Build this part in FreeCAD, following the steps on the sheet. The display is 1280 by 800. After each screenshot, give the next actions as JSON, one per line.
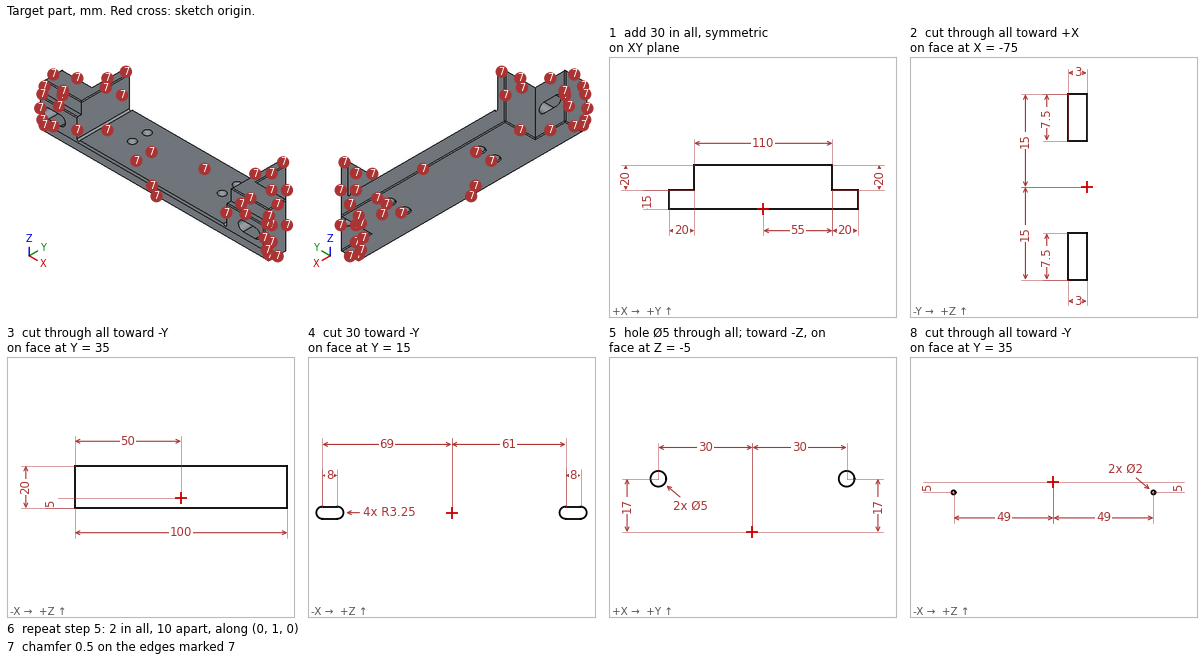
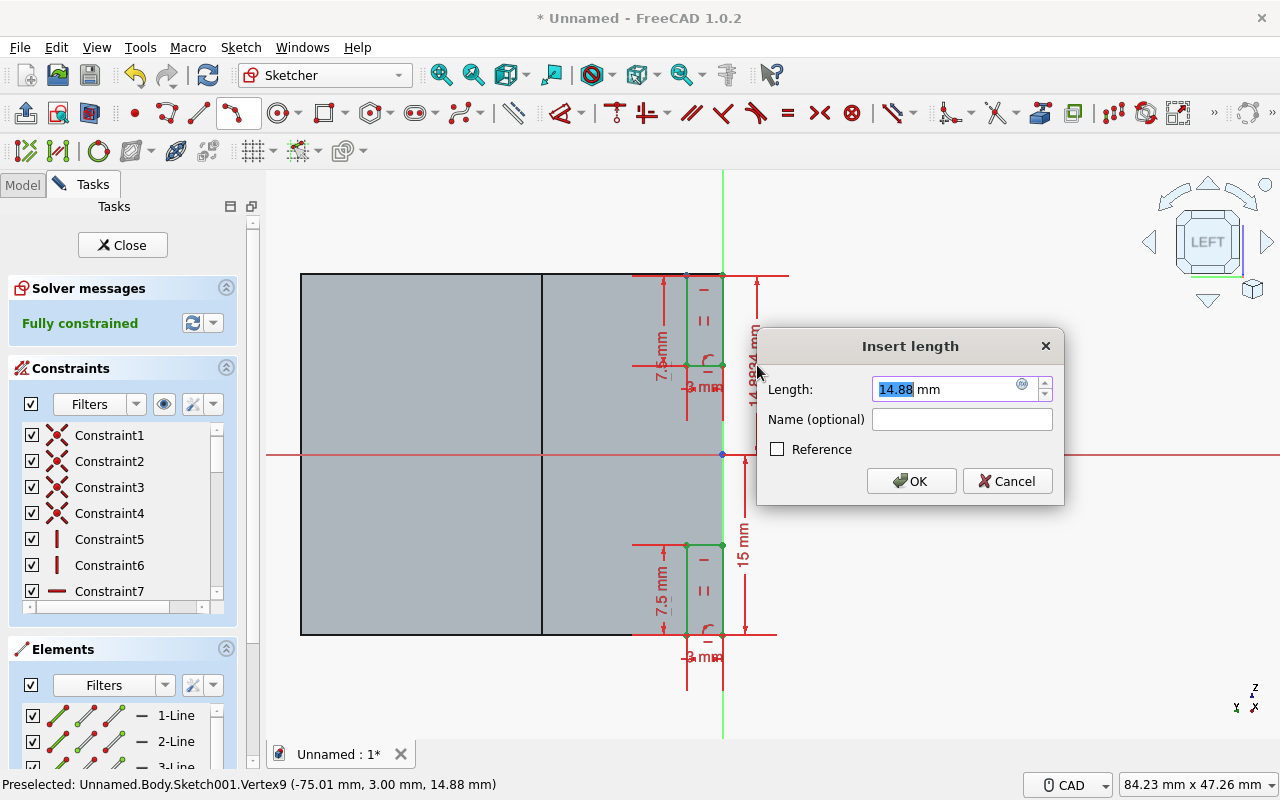
{"action": "type", "text": "15"}
{"action": "key", "text": "Return"}
{"action": "key", "text": "Escape"}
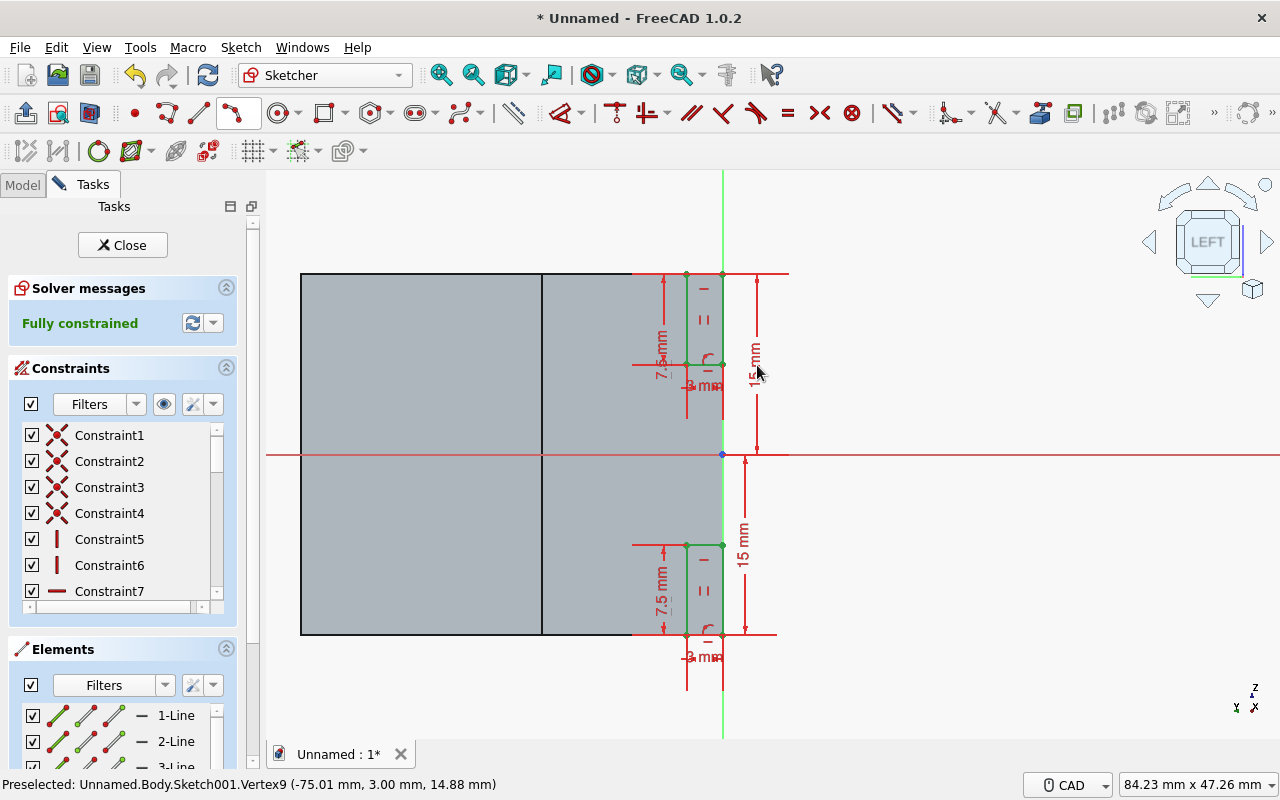
{"action": "left_click", "coordinate": [123, 245]}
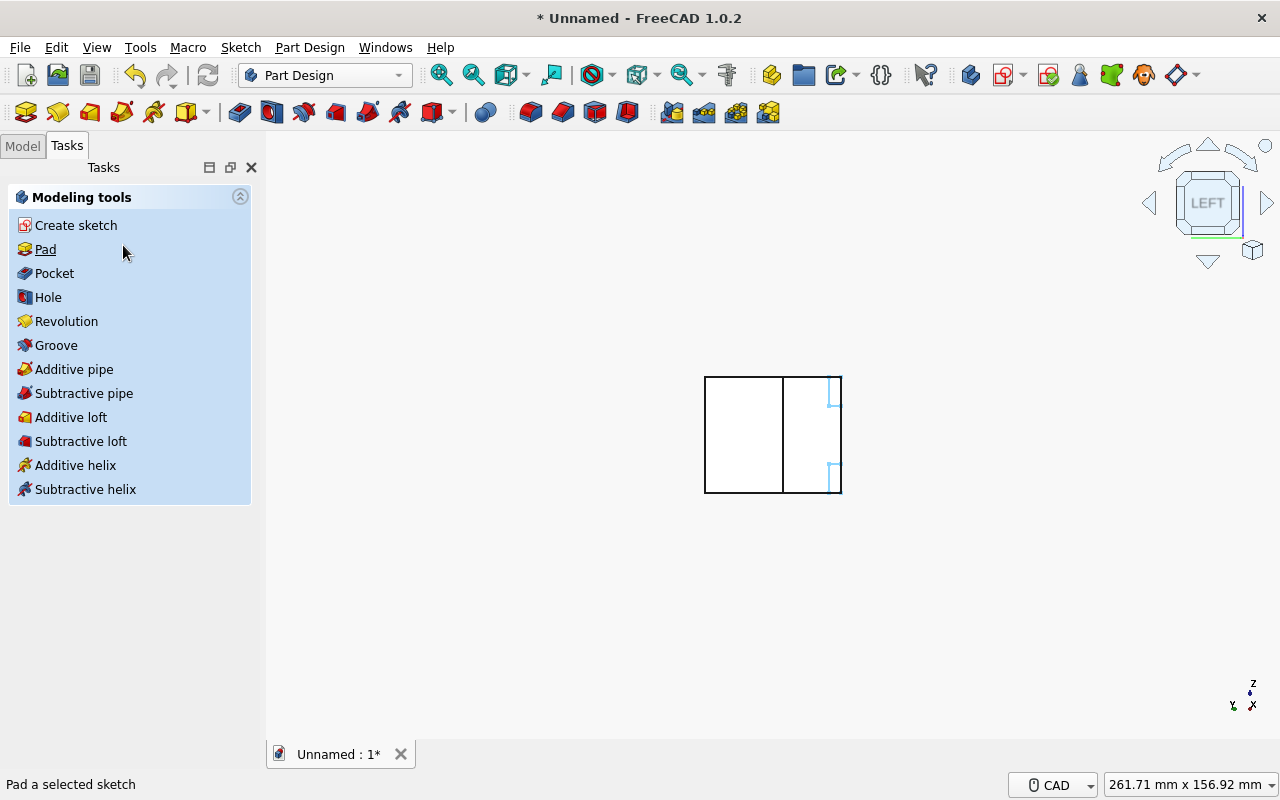
{"action": "left_click", "coordinate": [240, 112]}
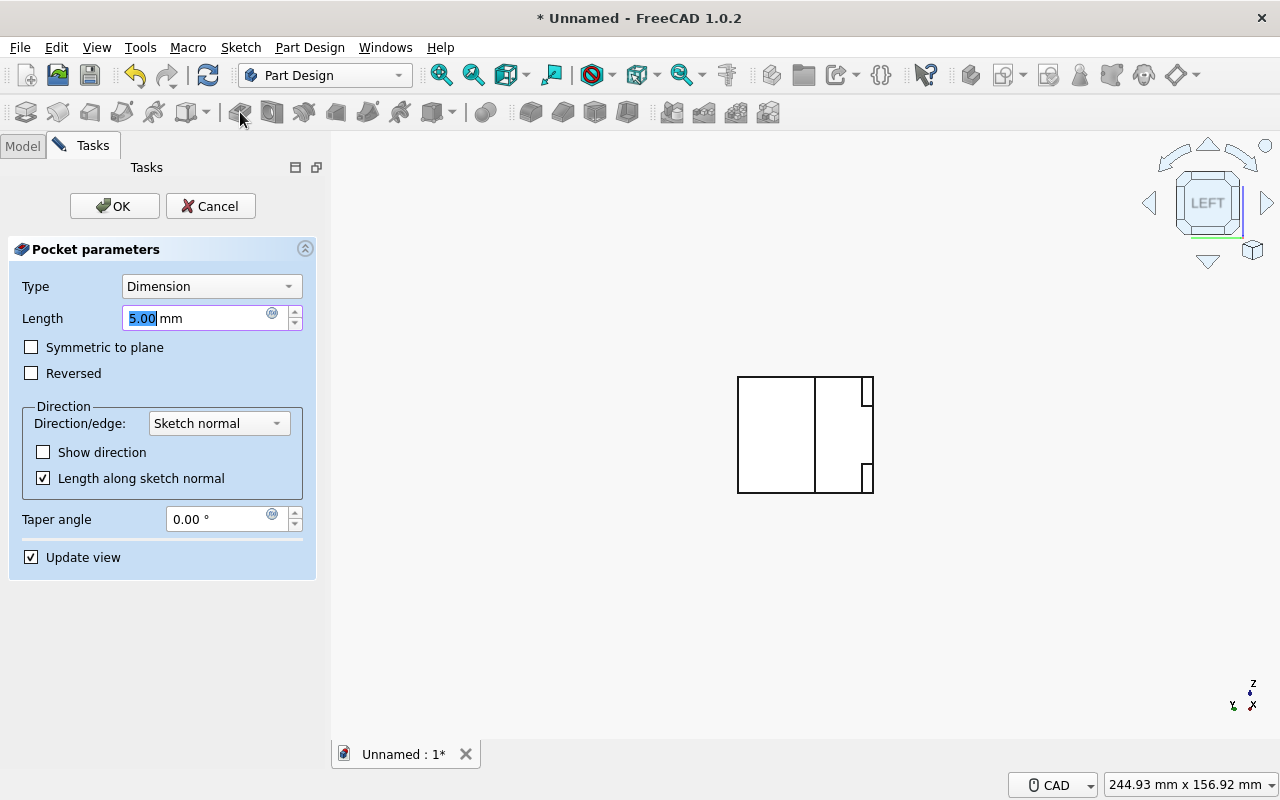
{"action": "left_click", "coordinate": [212, 286]}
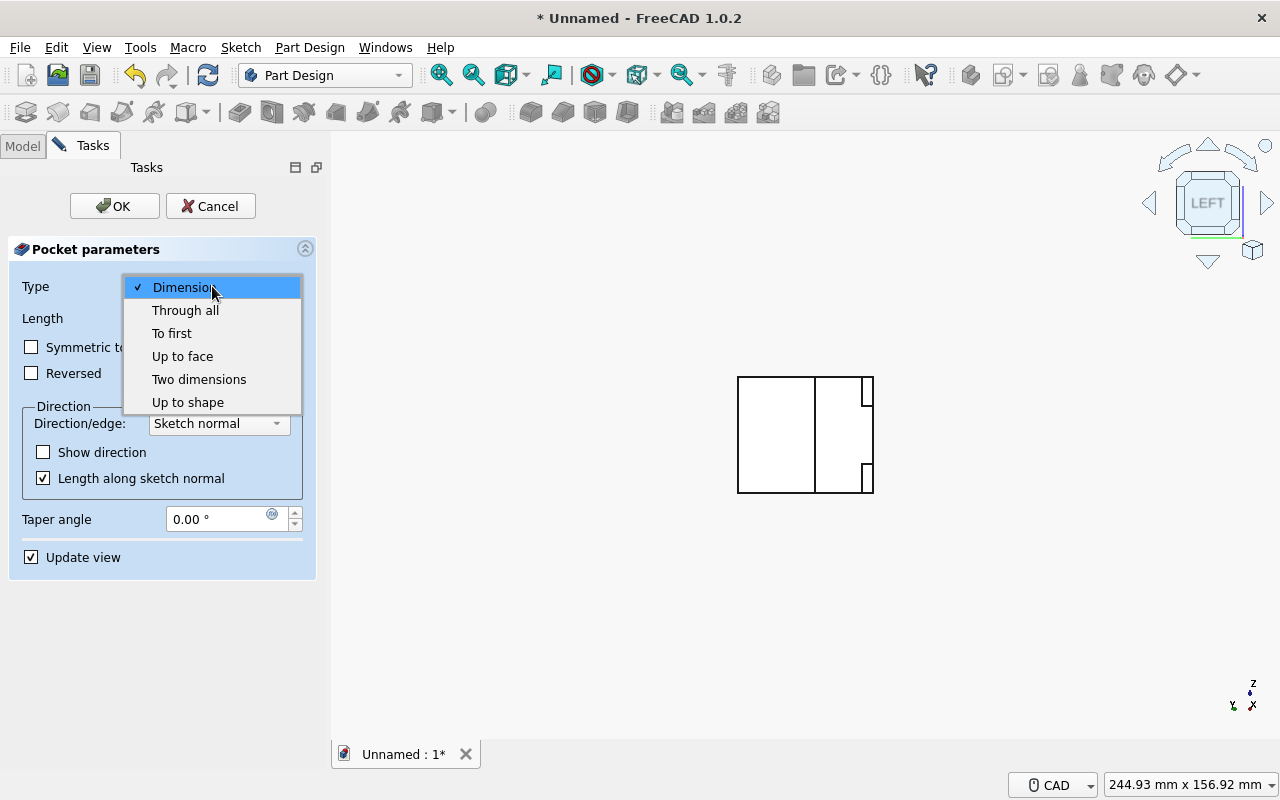
{"action": "left_click", "coordinate": [212, 310]}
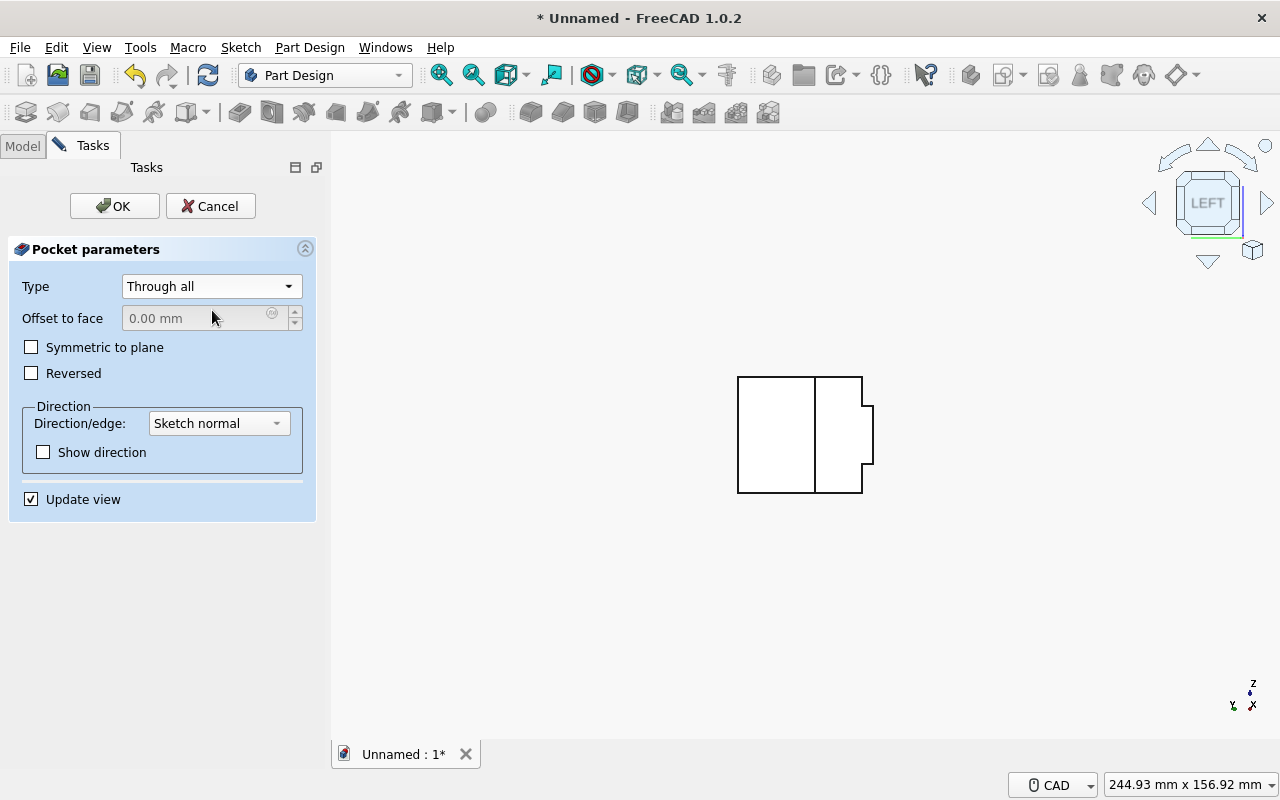
{"action": "left_click", "coordinate": [115, 206]}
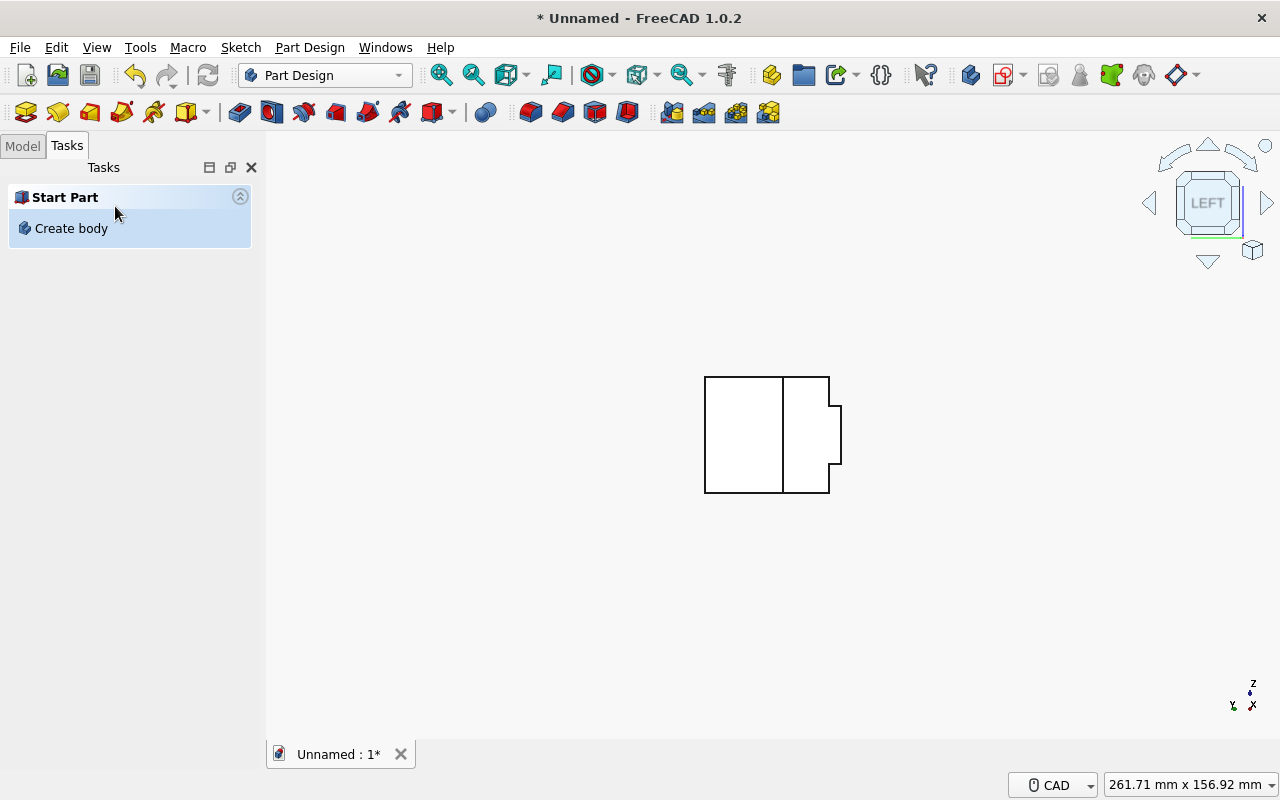
{"action": "left_click", "coordinate": [442, 76]}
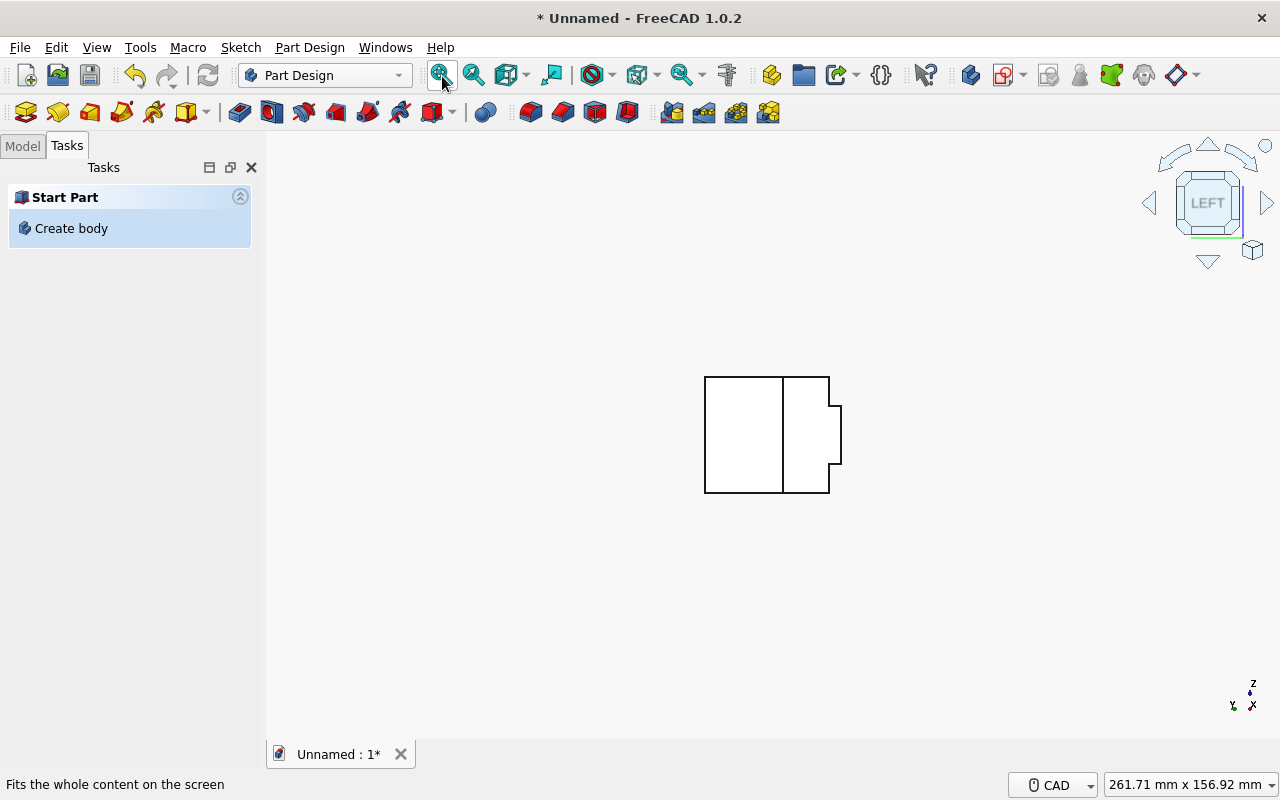
{"action": "key", "text": "4"}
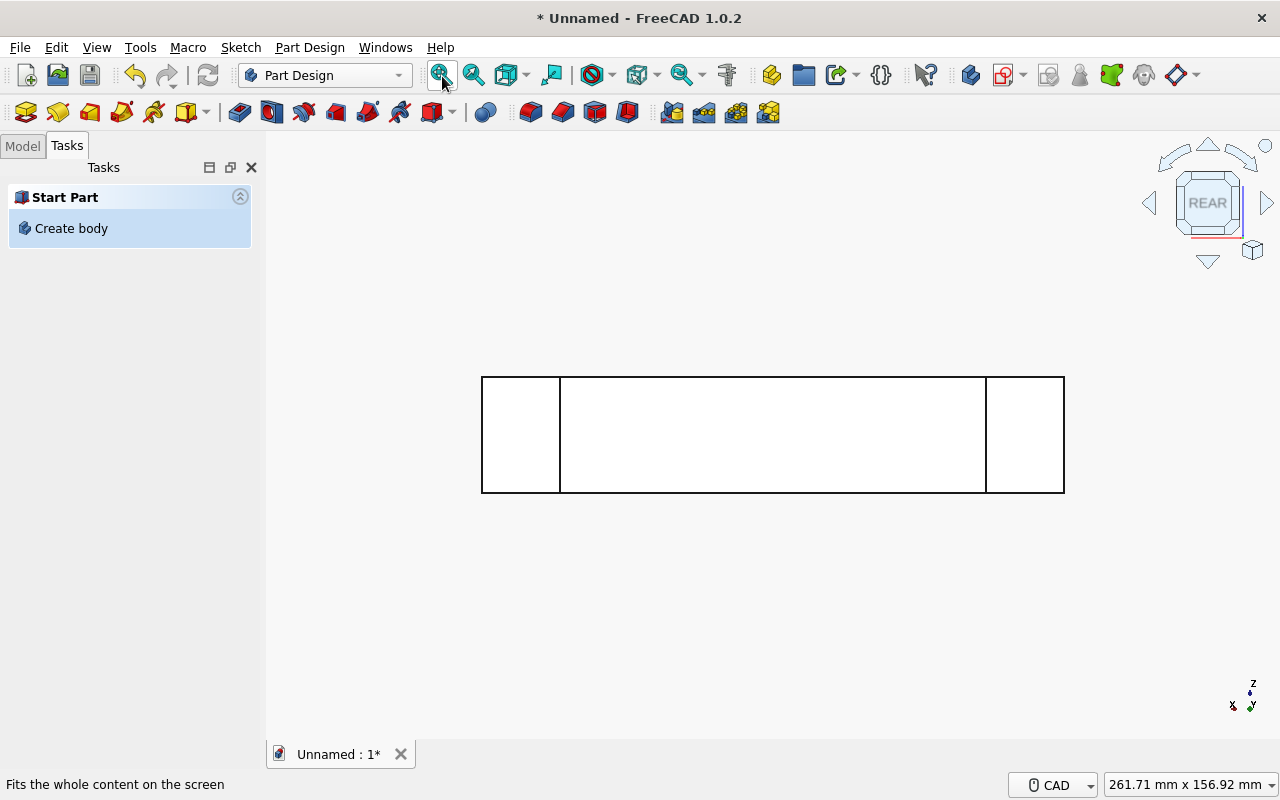
{"action": "left_click", "coordinate": [651, 434]}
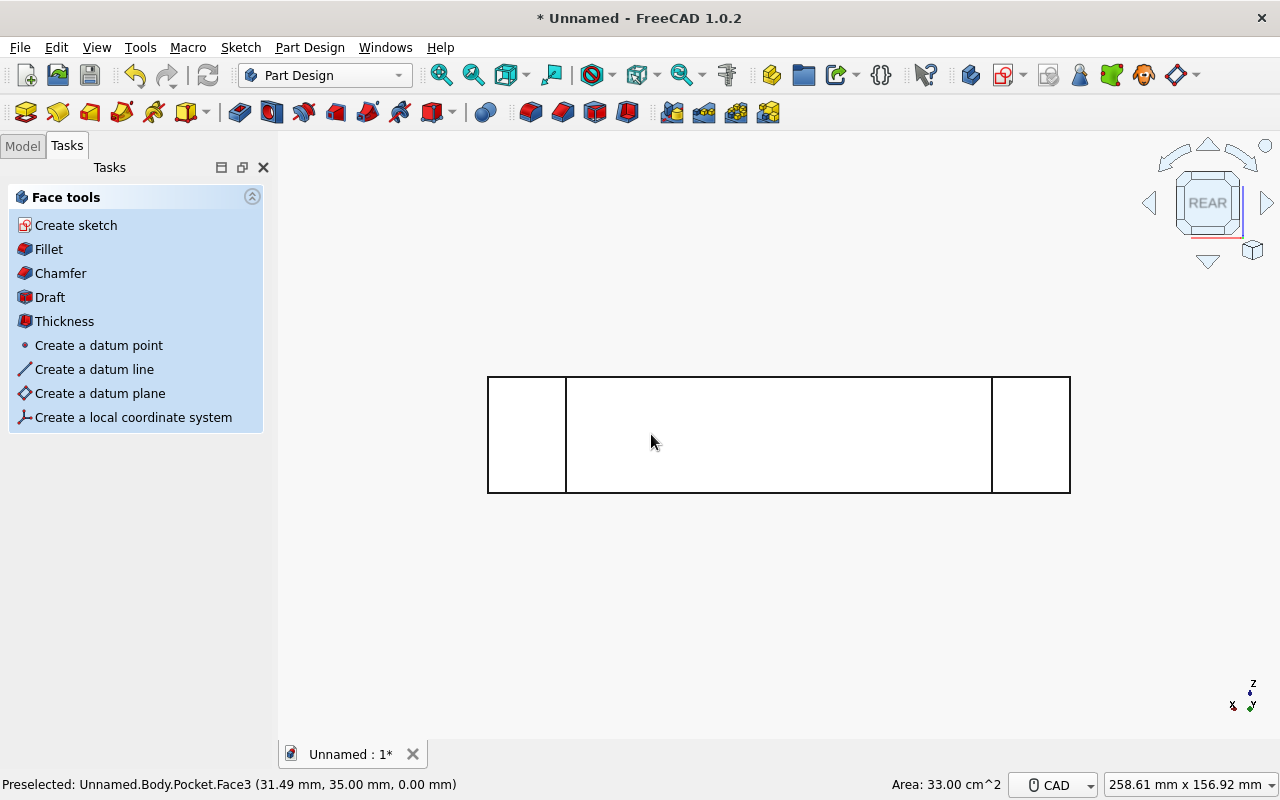
{"action": "left_click", "coordinate": [1004, 76]}